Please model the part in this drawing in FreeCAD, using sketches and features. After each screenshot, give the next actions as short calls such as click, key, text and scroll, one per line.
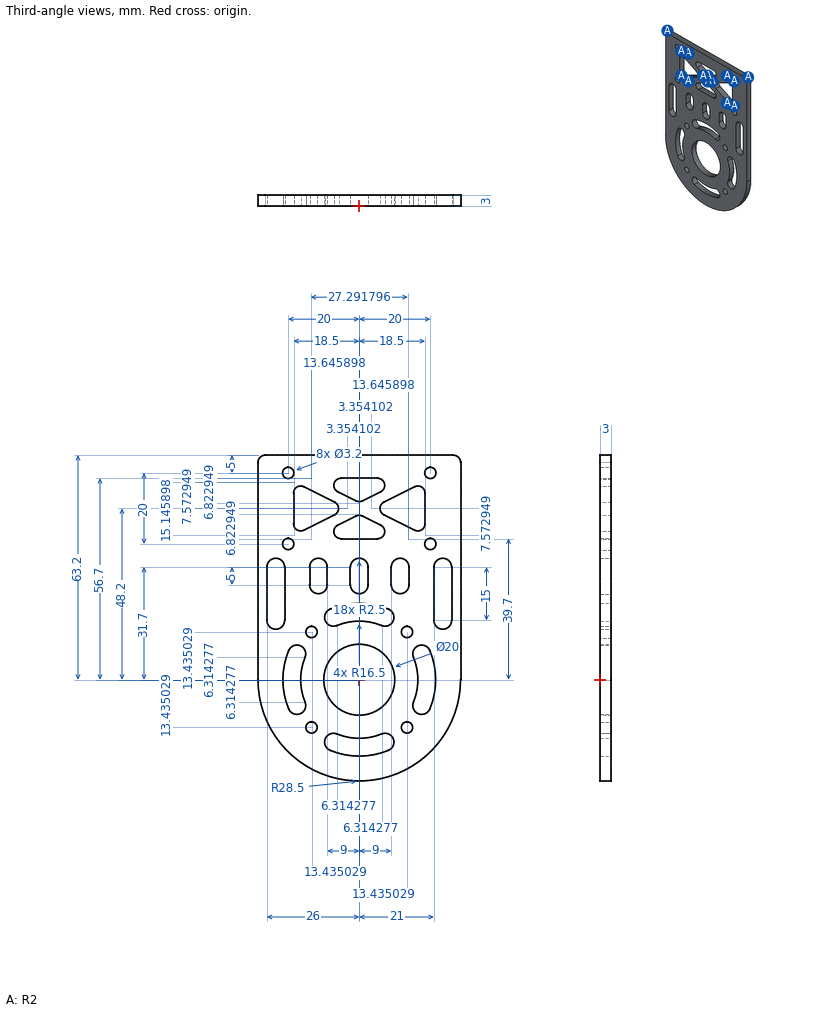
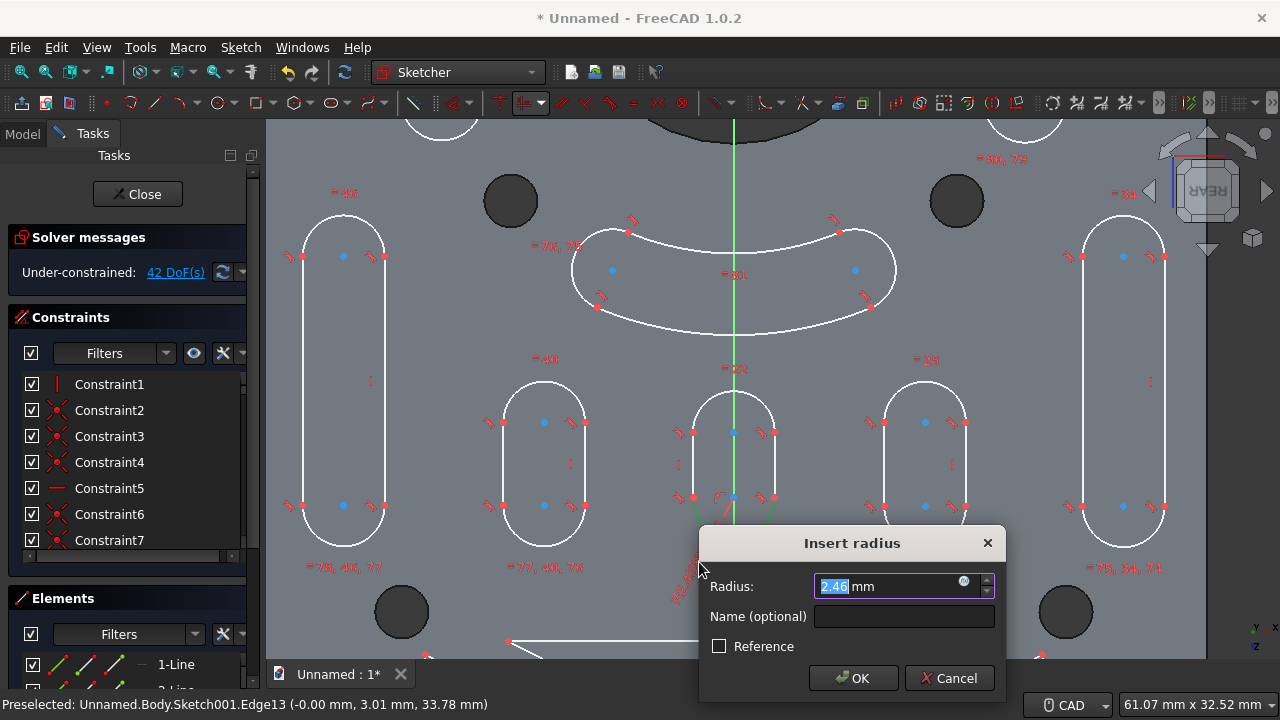
text(2.5)
key(Return)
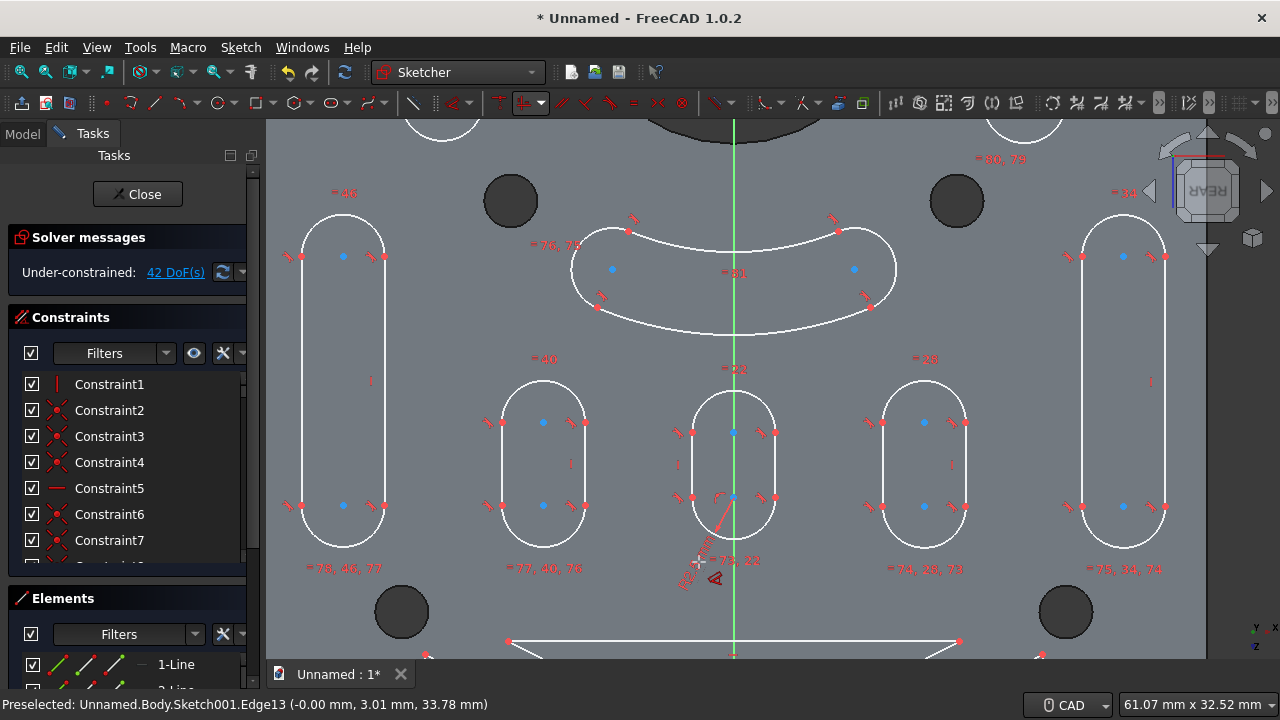
click(691, 249)
click(686, 281)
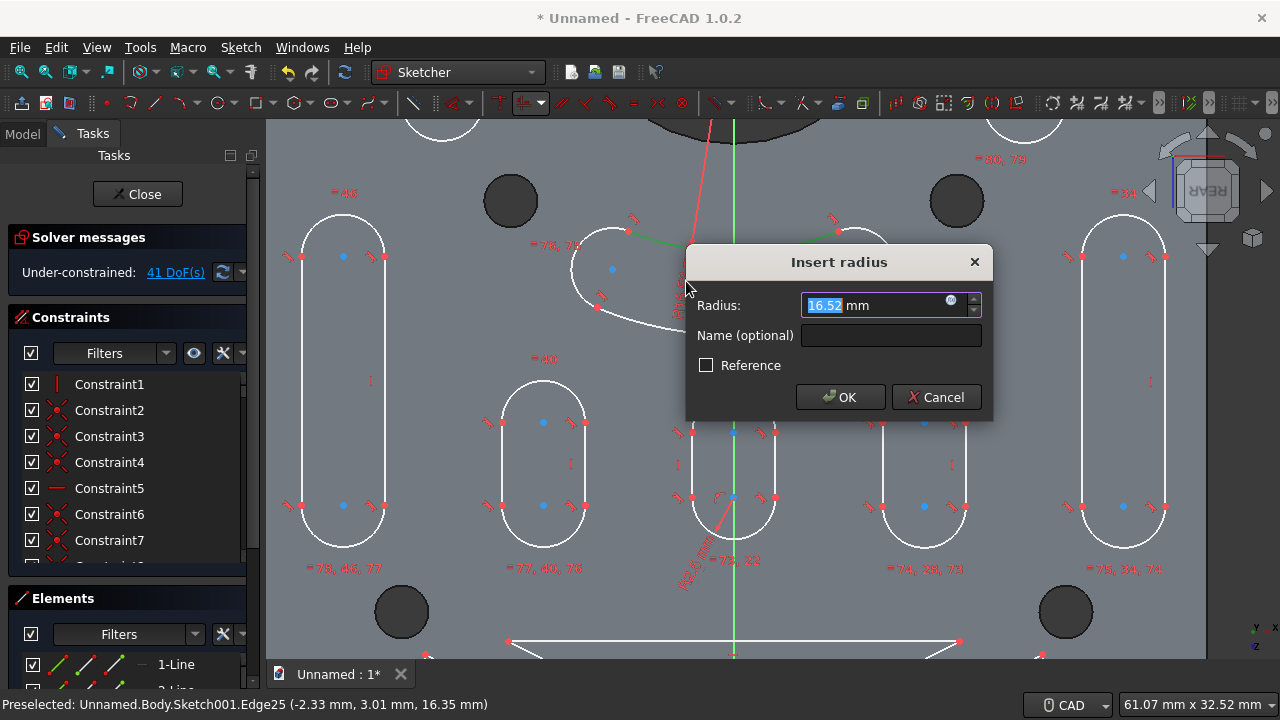
text(16.5)
key(Return)
key(Escape)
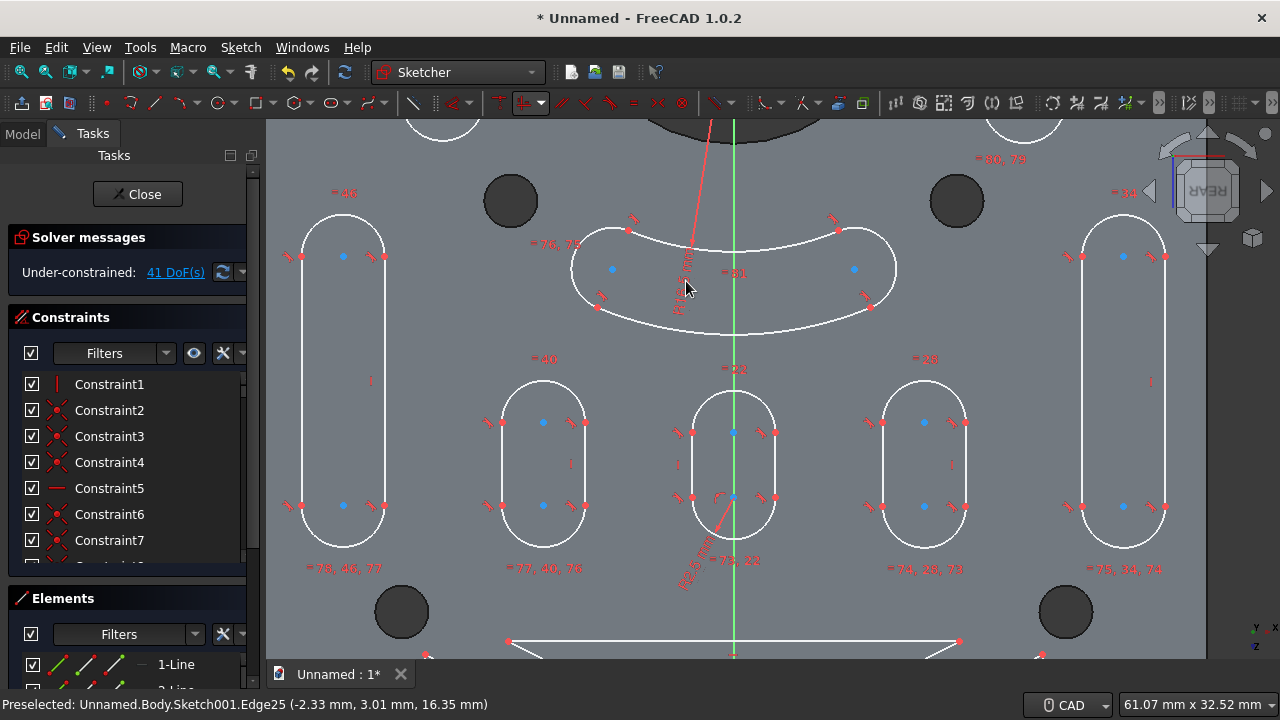
scroll(695, 428, down, 7)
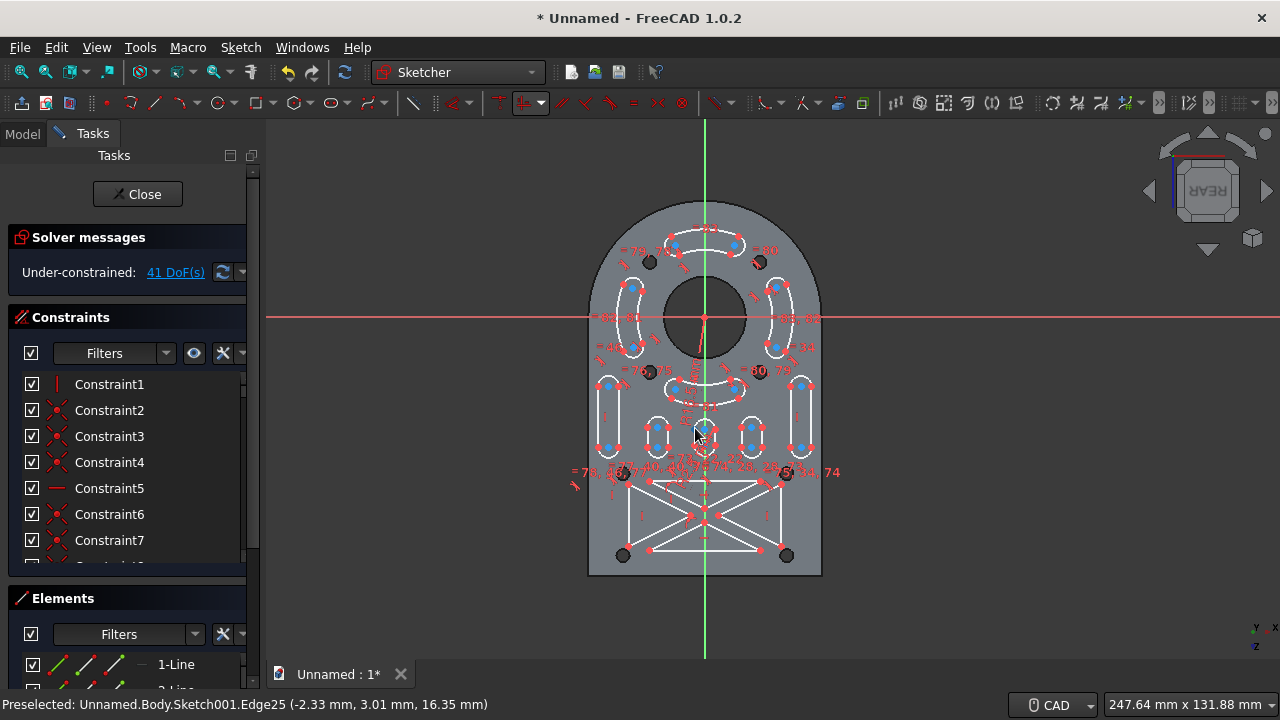
click(705, 509)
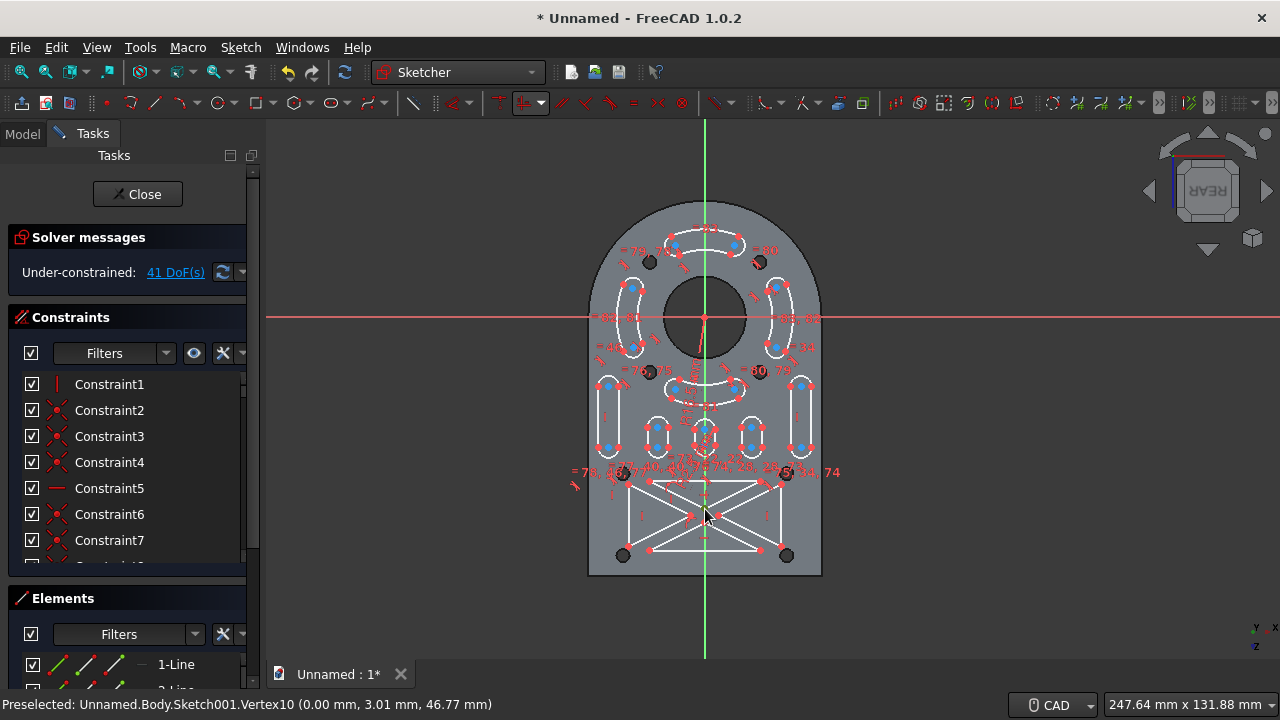
click(705, 596)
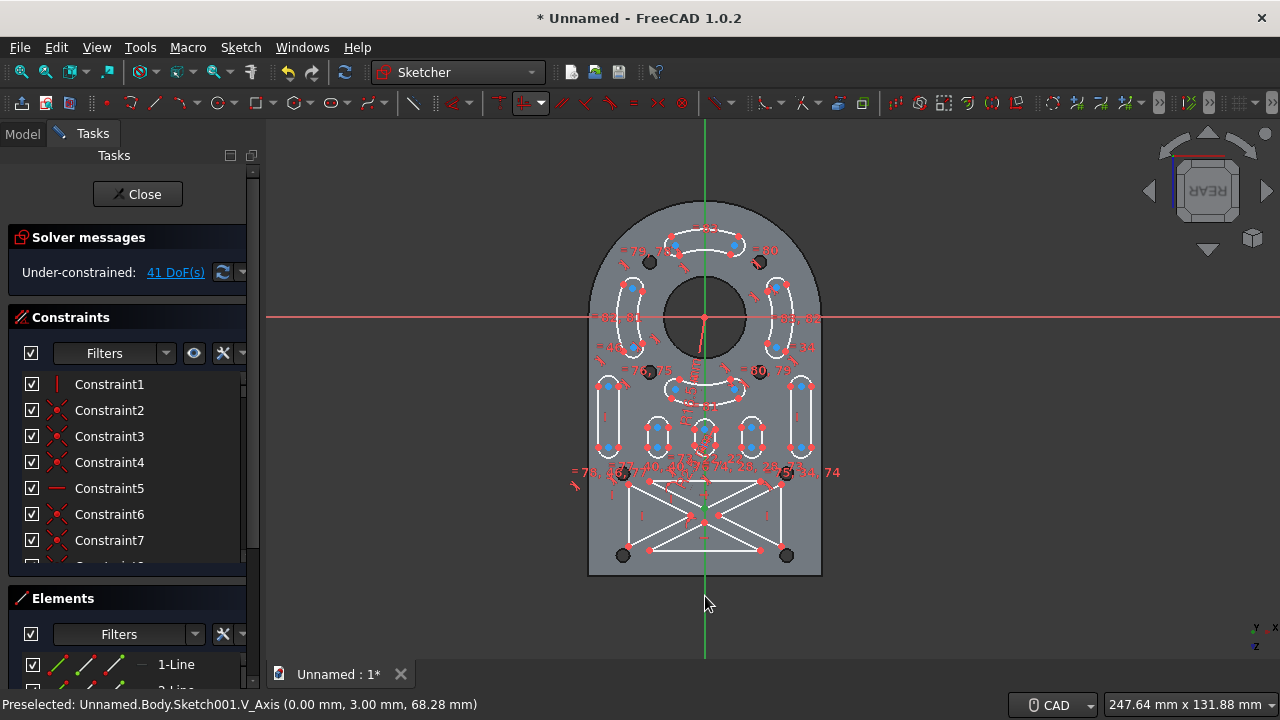
key(c)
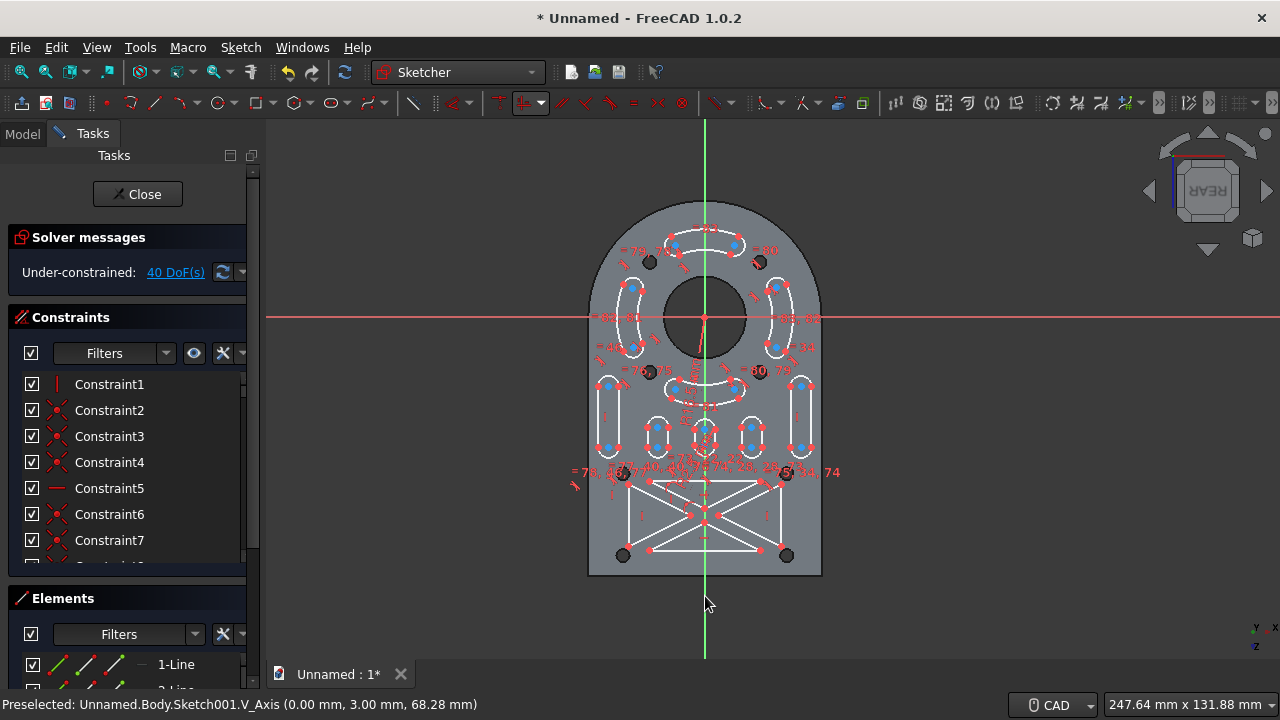
key(d)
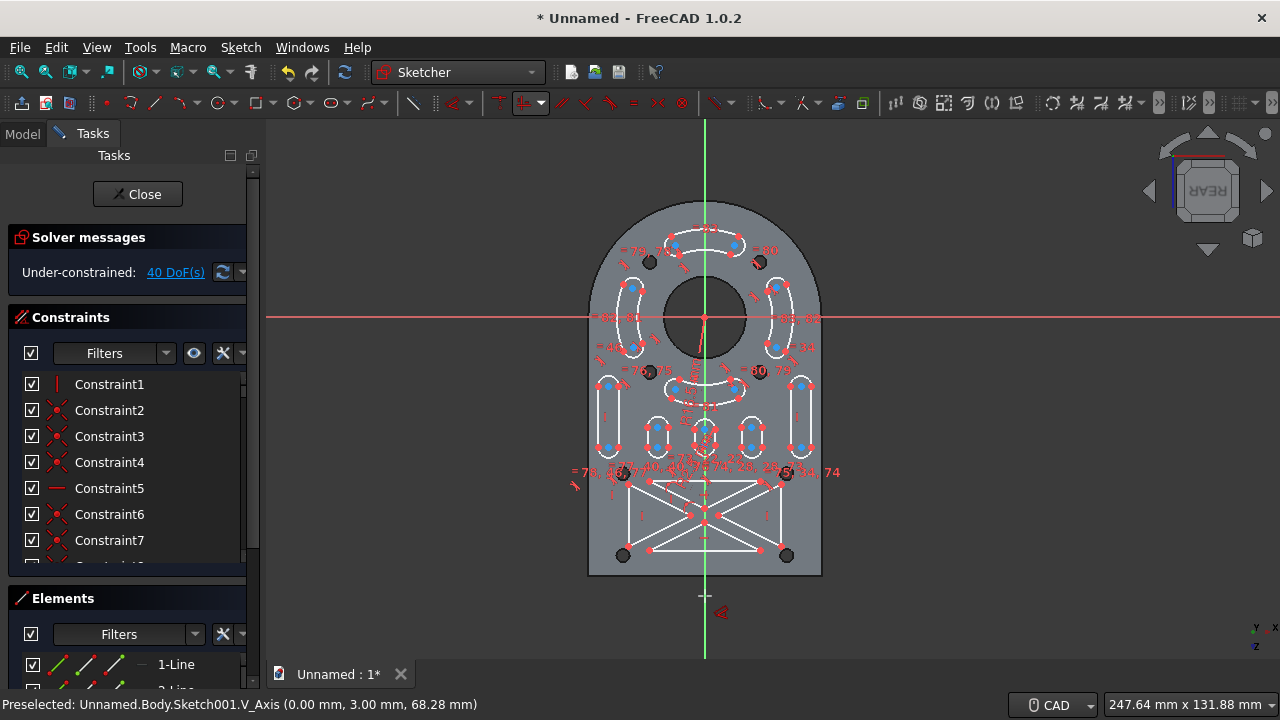
scroll(695, 438, up, 4)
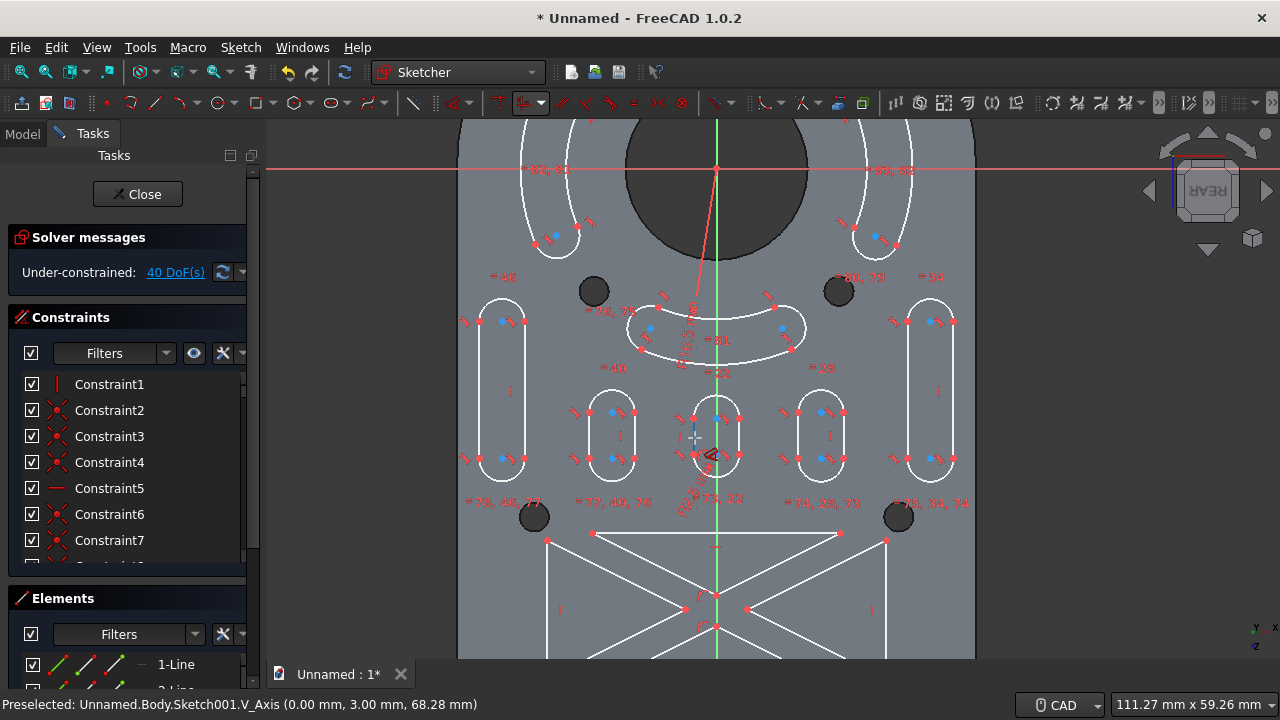
click(694, 436)
click(660, 436)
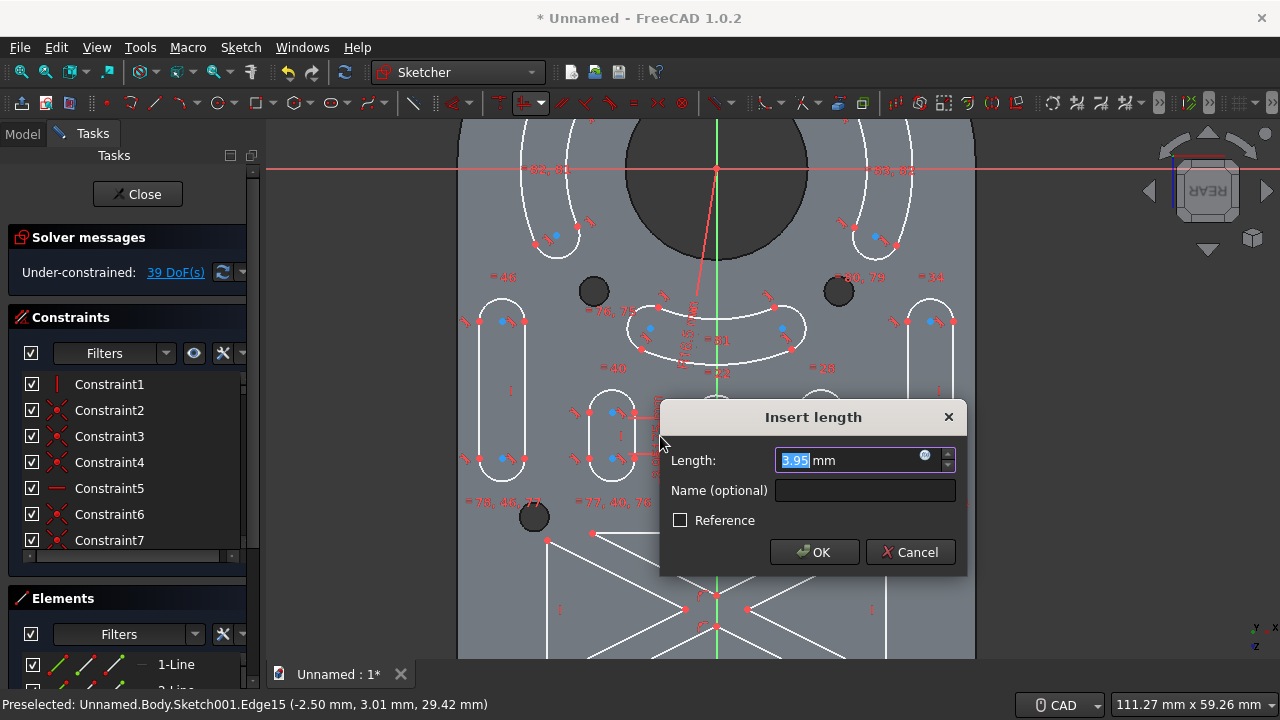
text(5)
key(Return)